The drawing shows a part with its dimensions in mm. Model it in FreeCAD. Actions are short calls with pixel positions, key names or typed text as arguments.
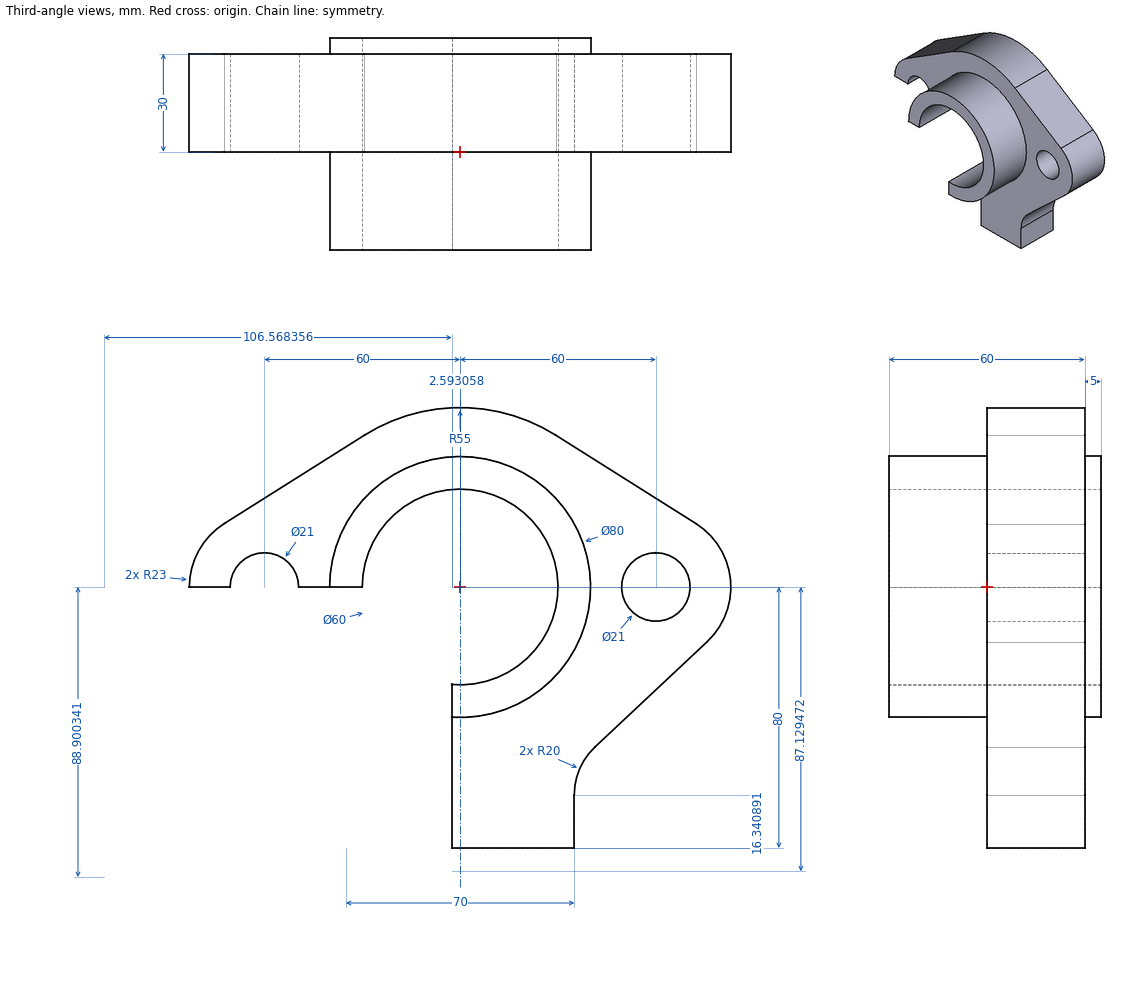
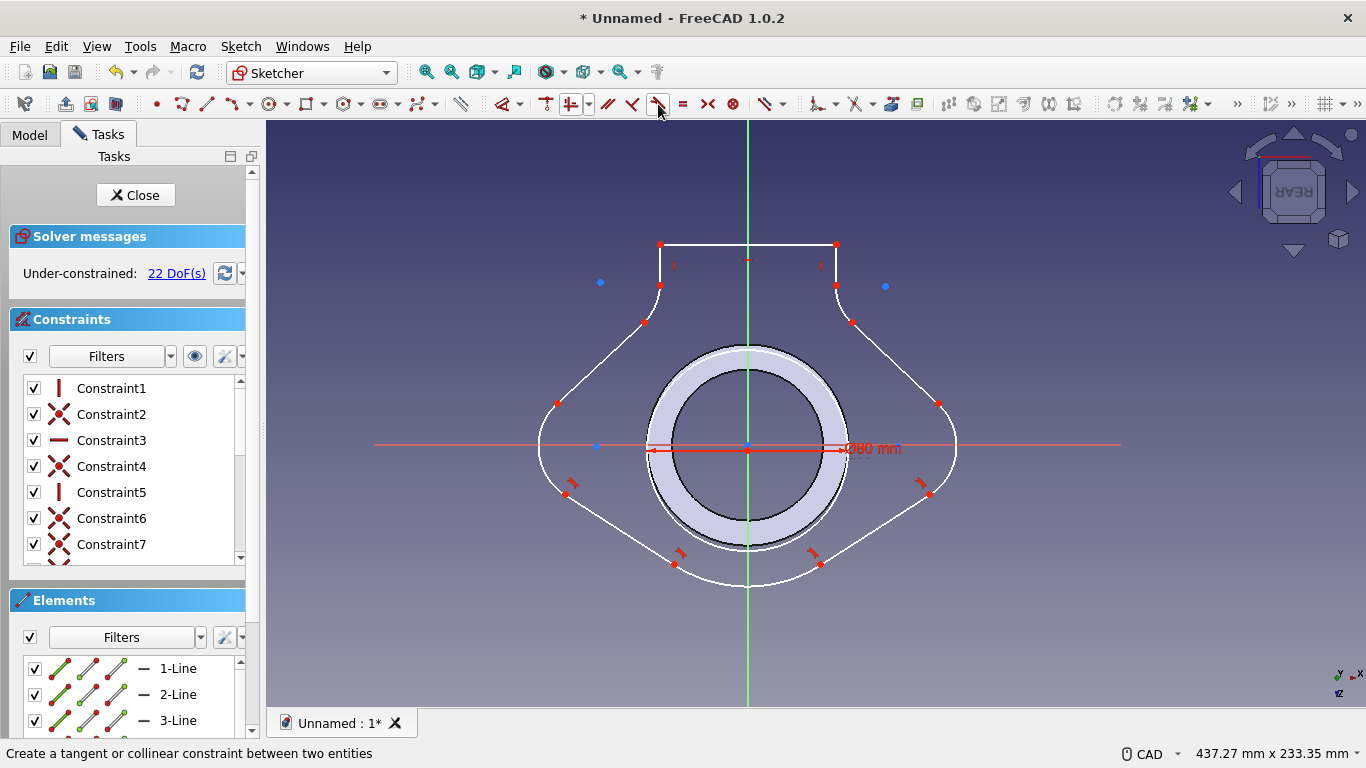
click(912, 380)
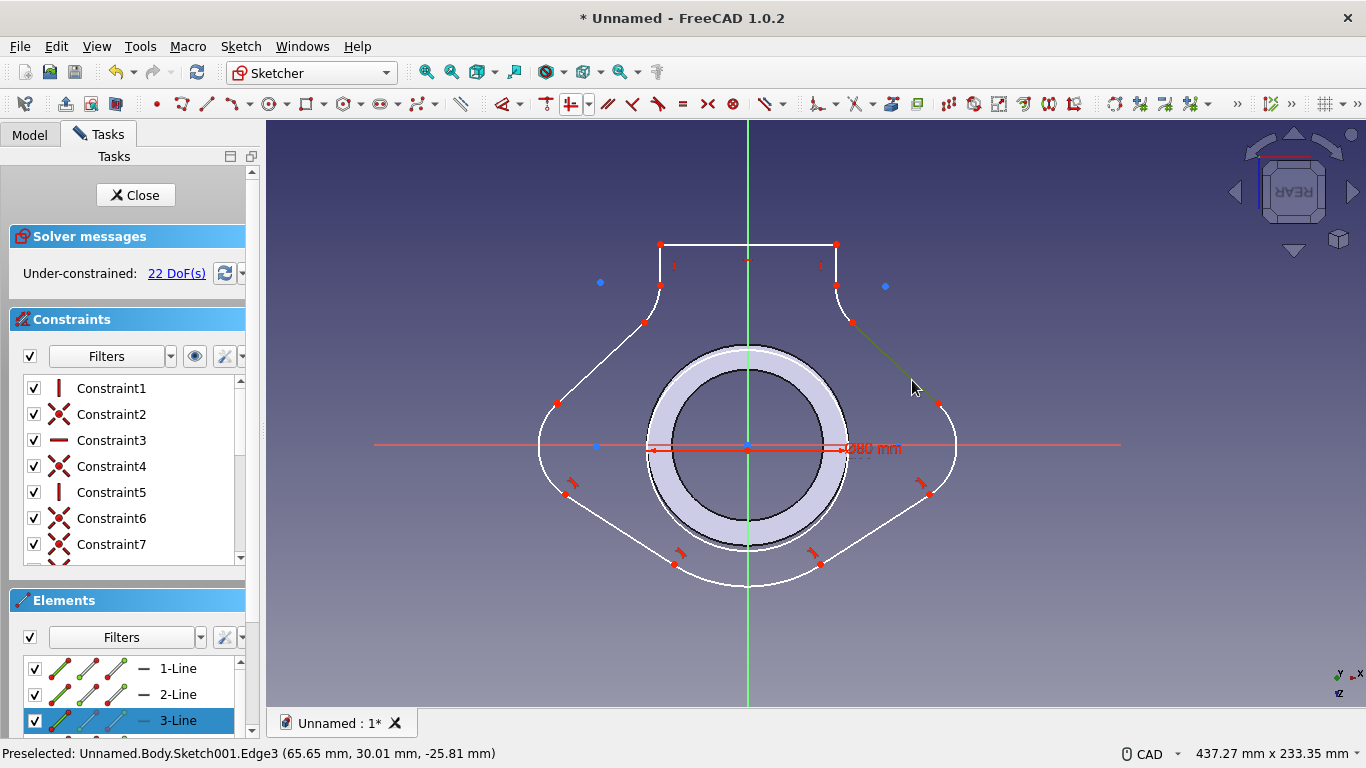
click(951, 472)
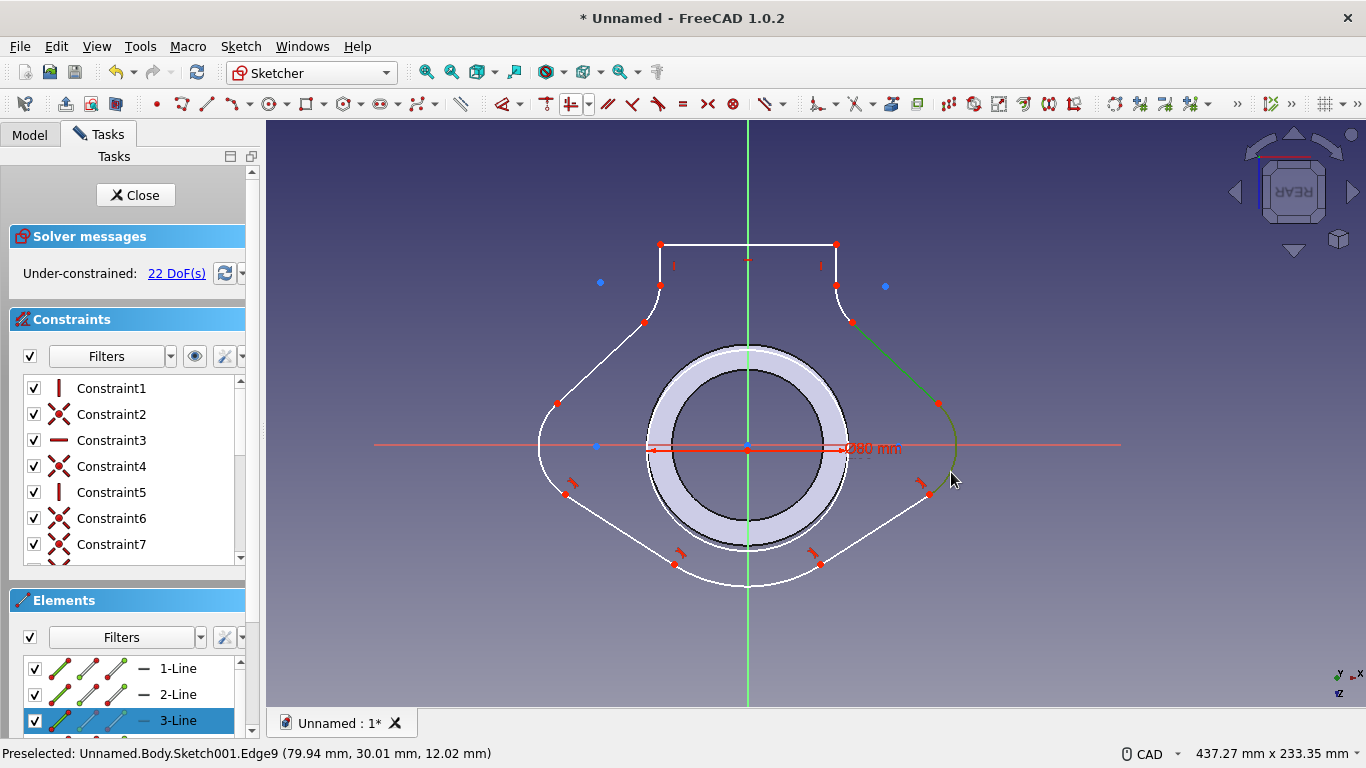
click(658, 104)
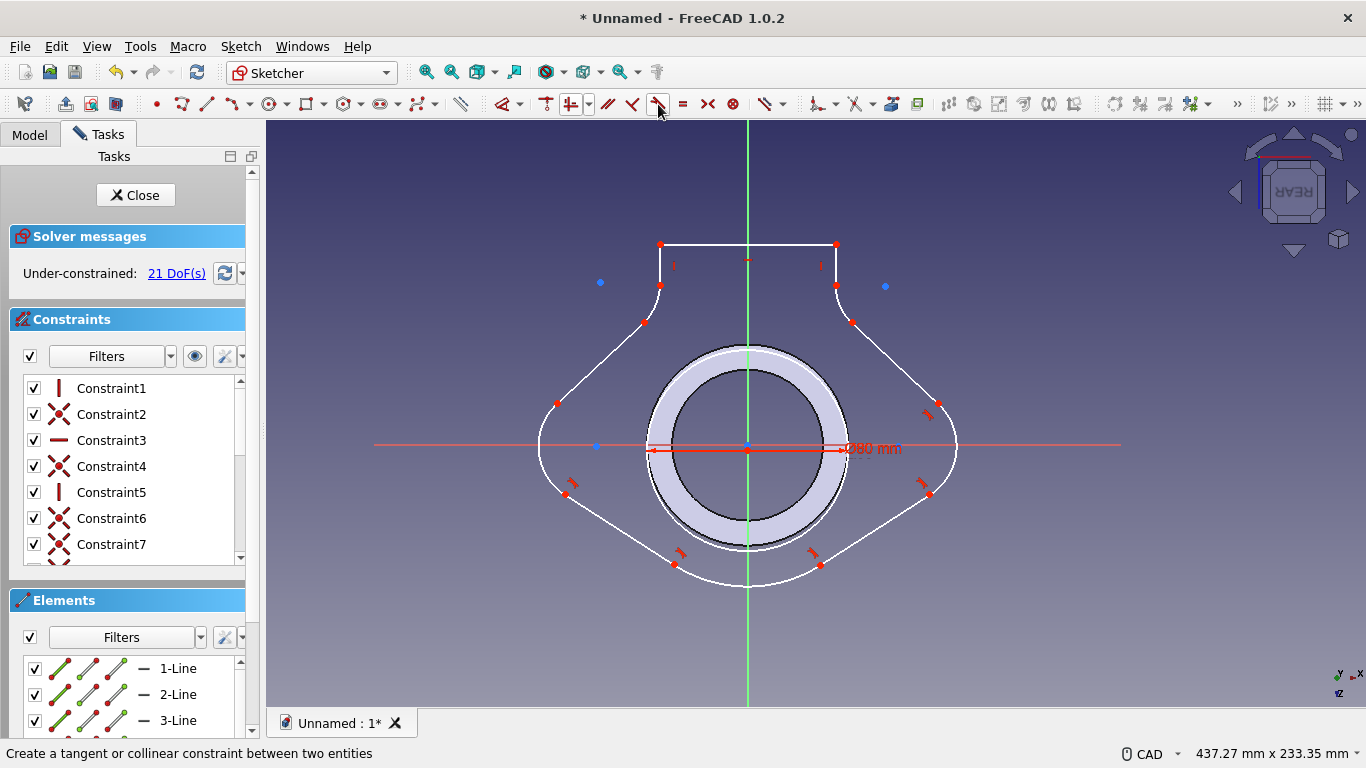
click(912, 380)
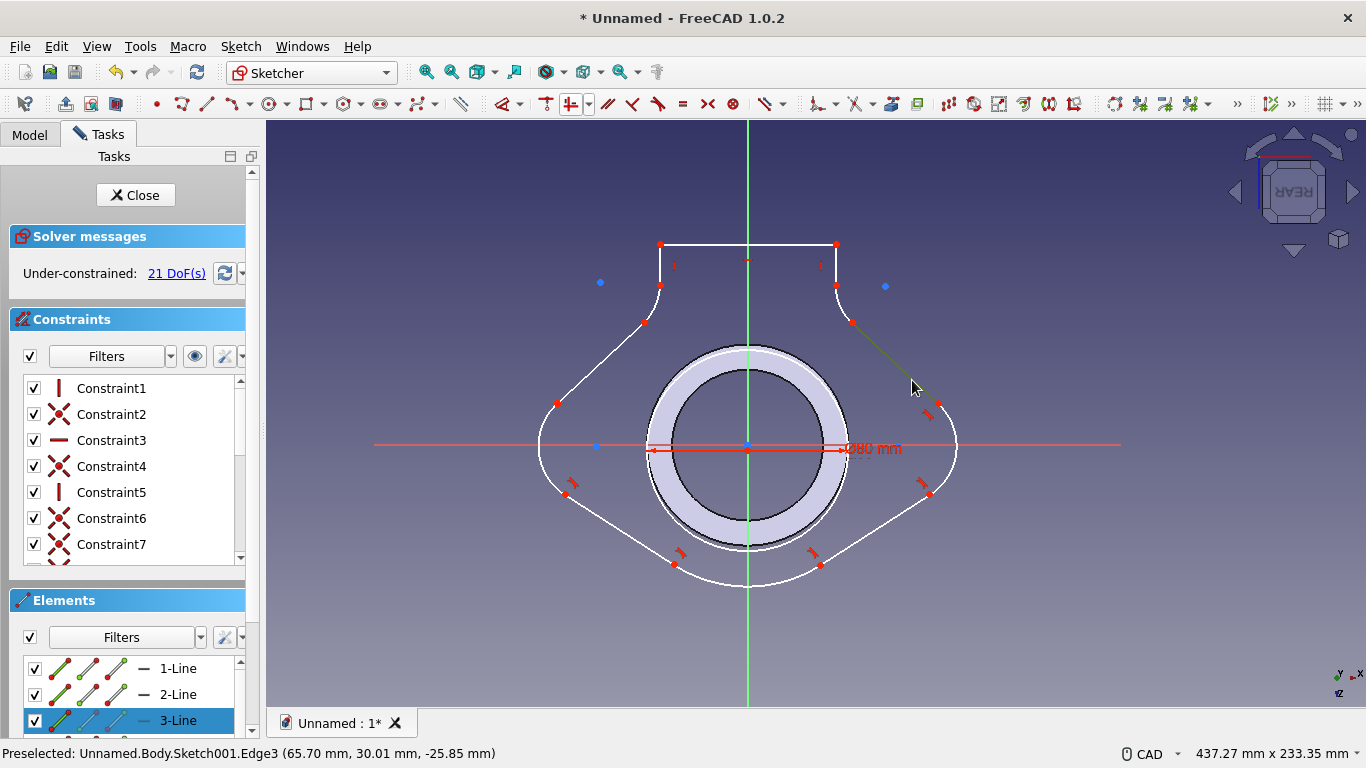
click(837, 298)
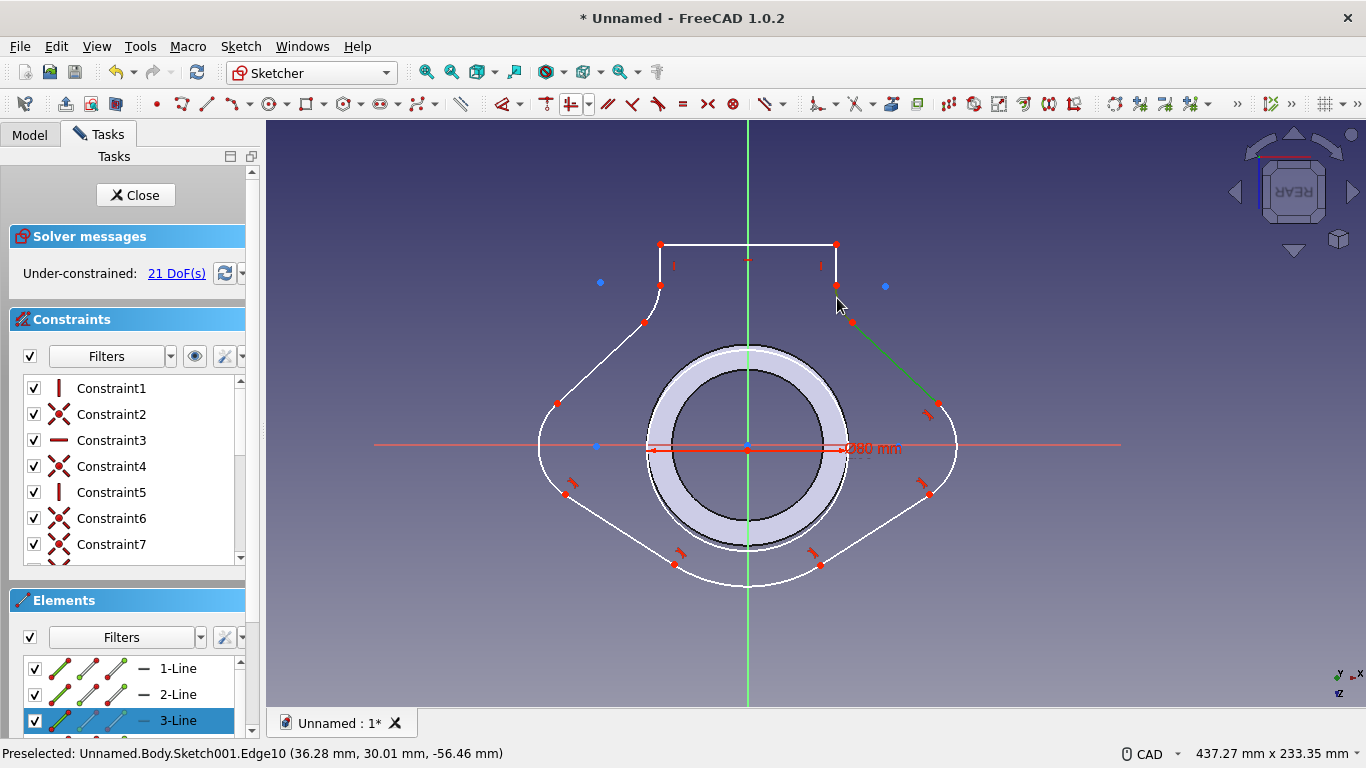
click(658, 104)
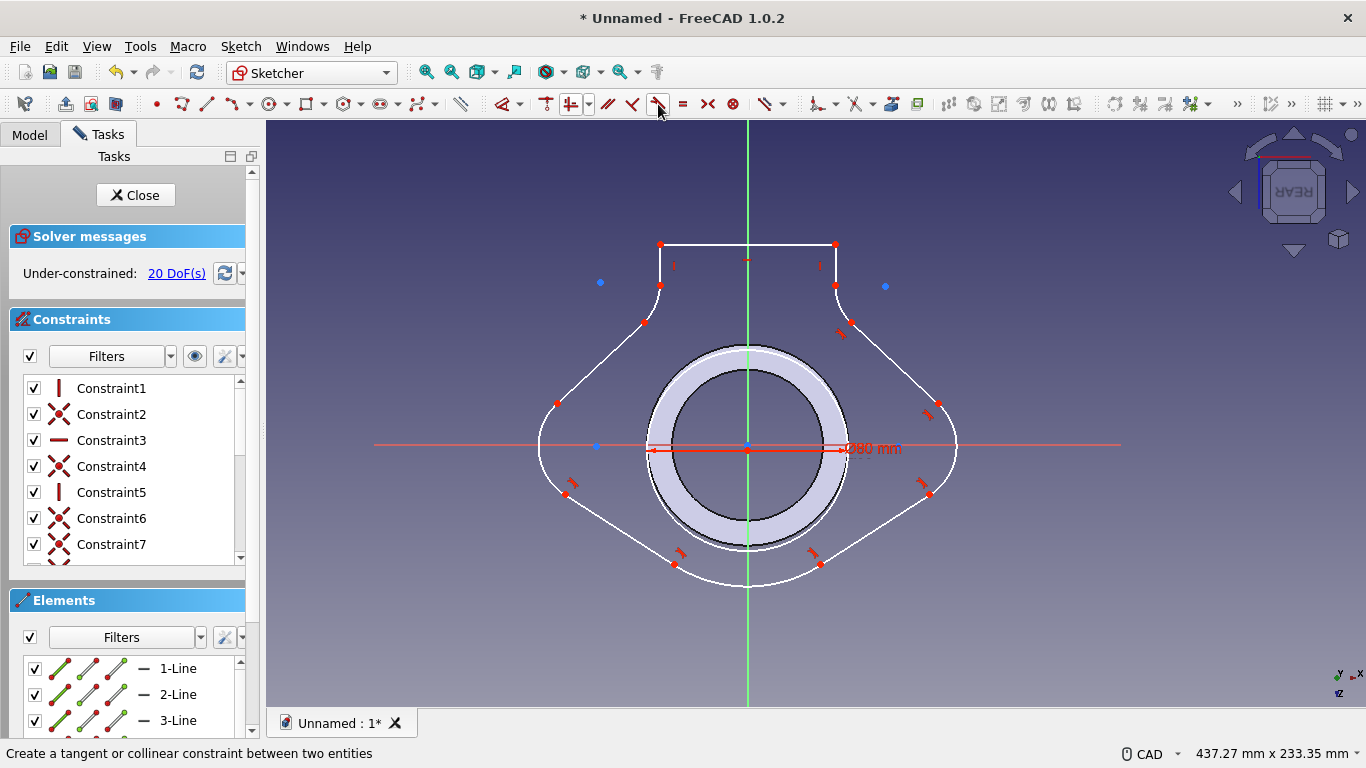
click(836, 274)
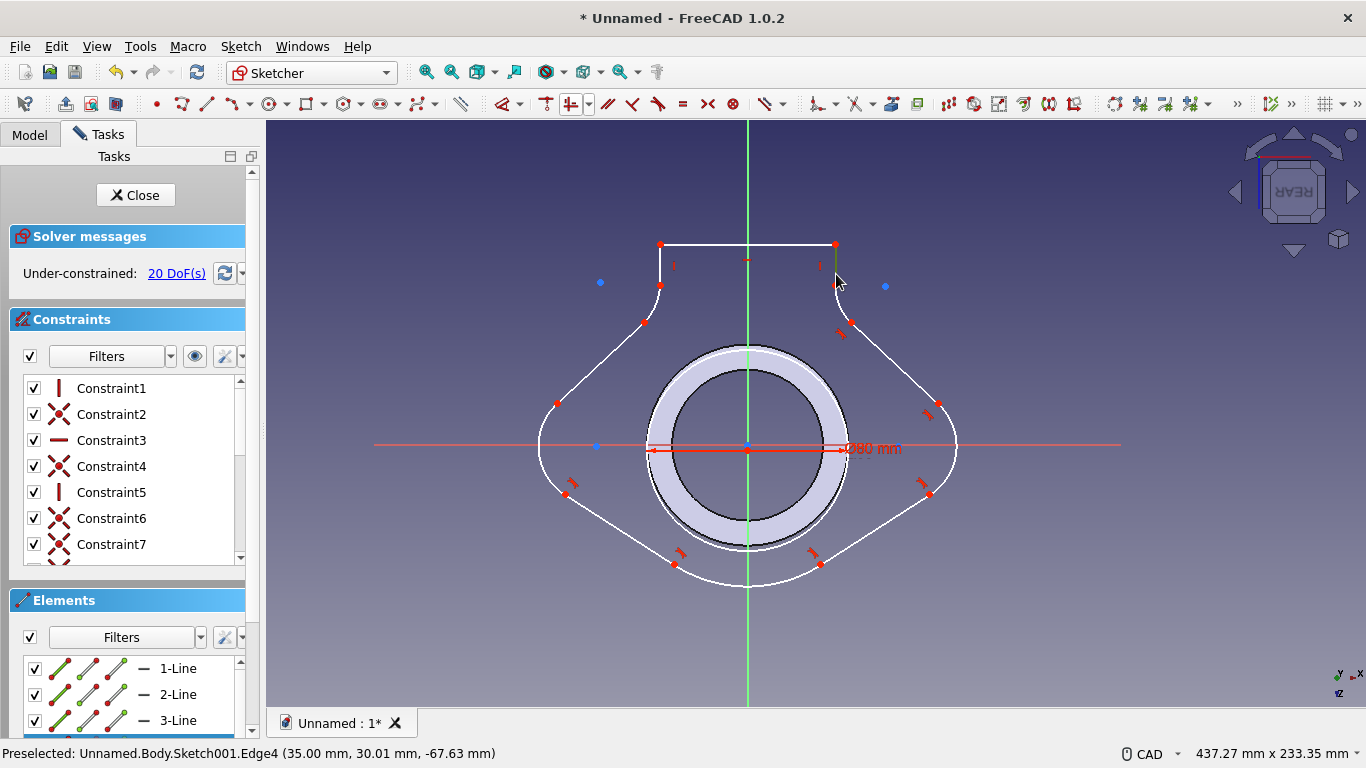
click(837, 298)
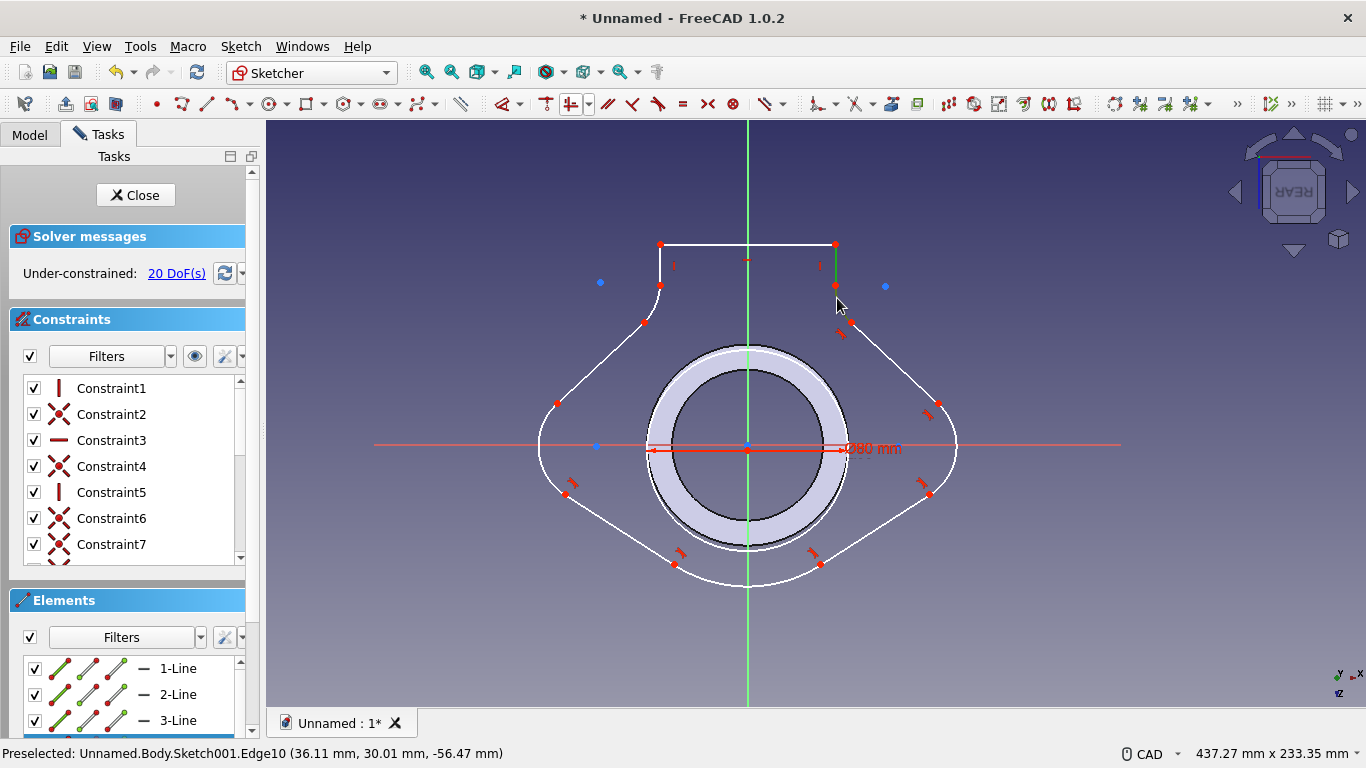
click(658, 104)